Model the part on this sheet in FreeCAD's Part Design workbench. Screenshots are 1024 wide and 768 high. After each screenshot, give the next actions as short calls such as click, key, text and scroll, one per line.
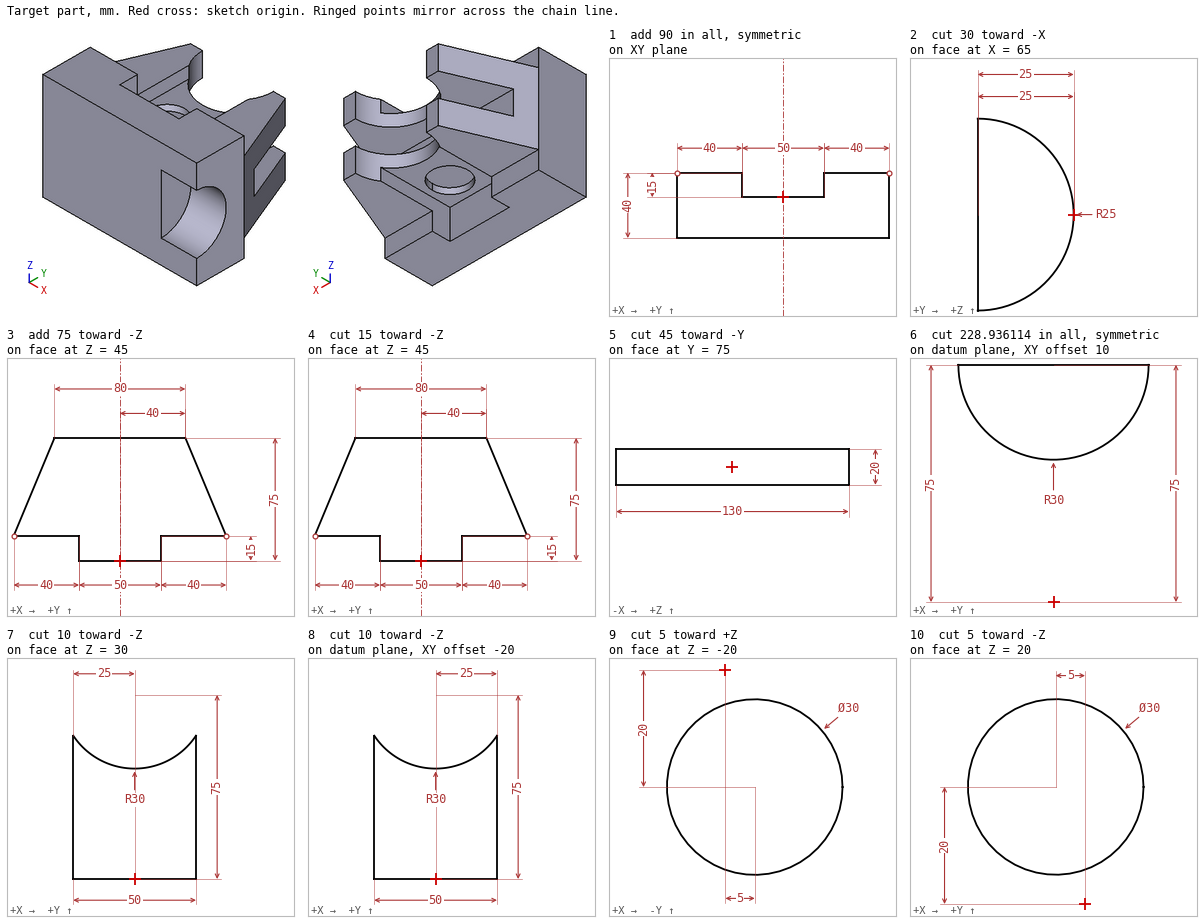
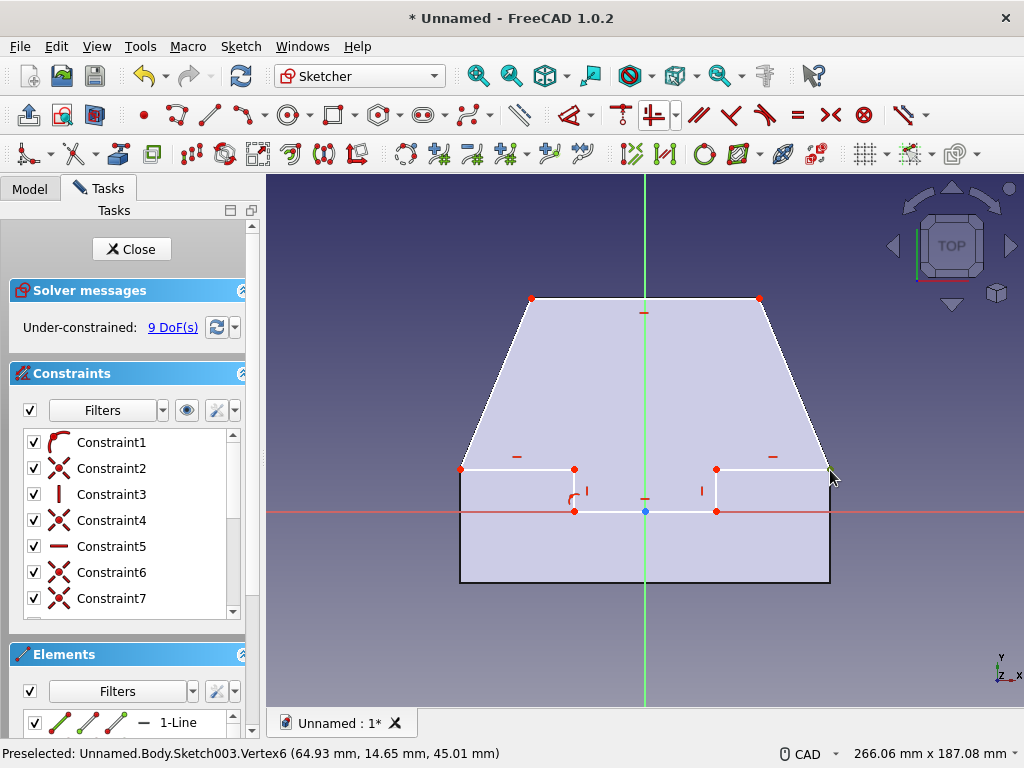
click(460, 470)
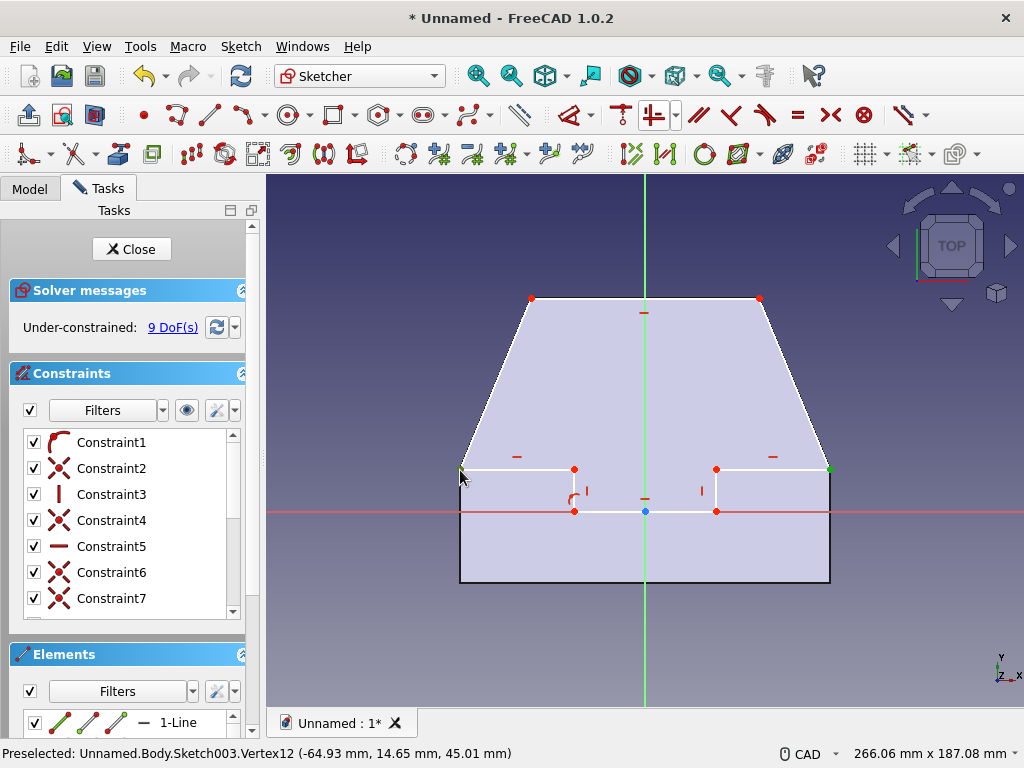
click(645, 645)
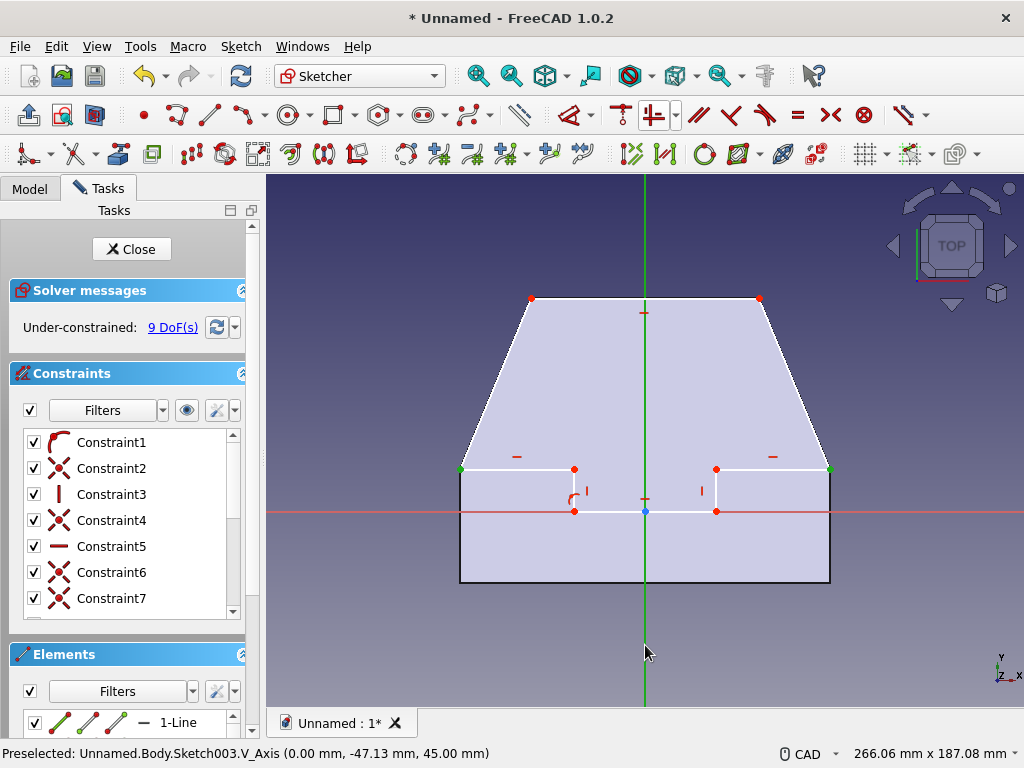
click(831, 116)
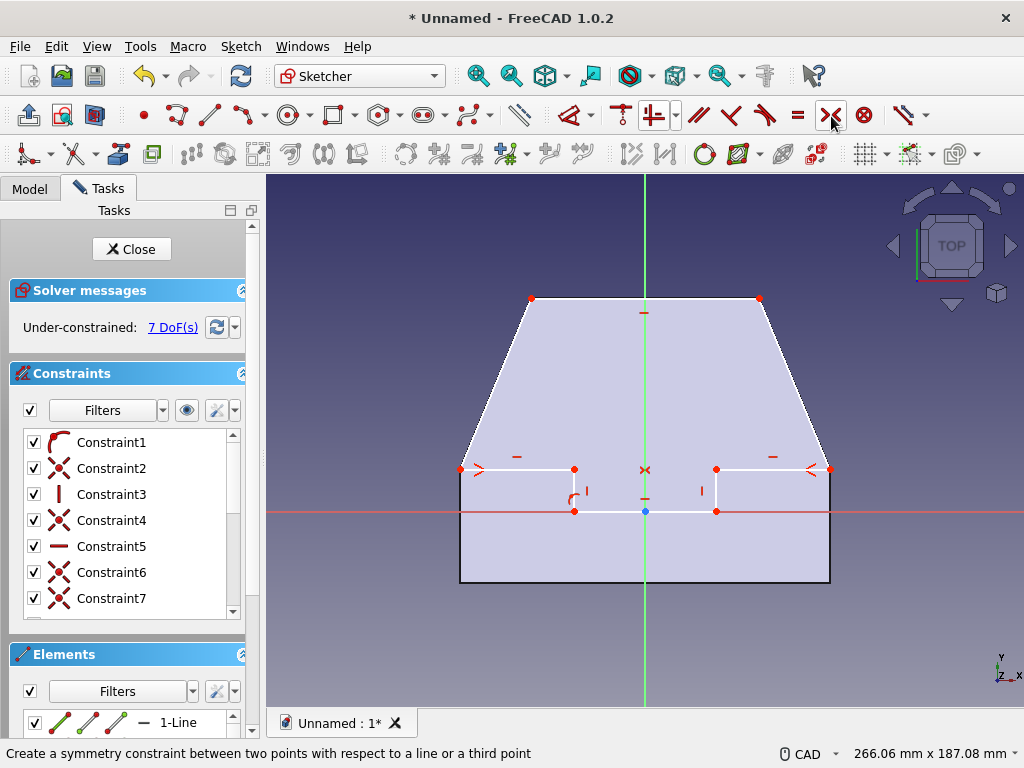
click(568, 116)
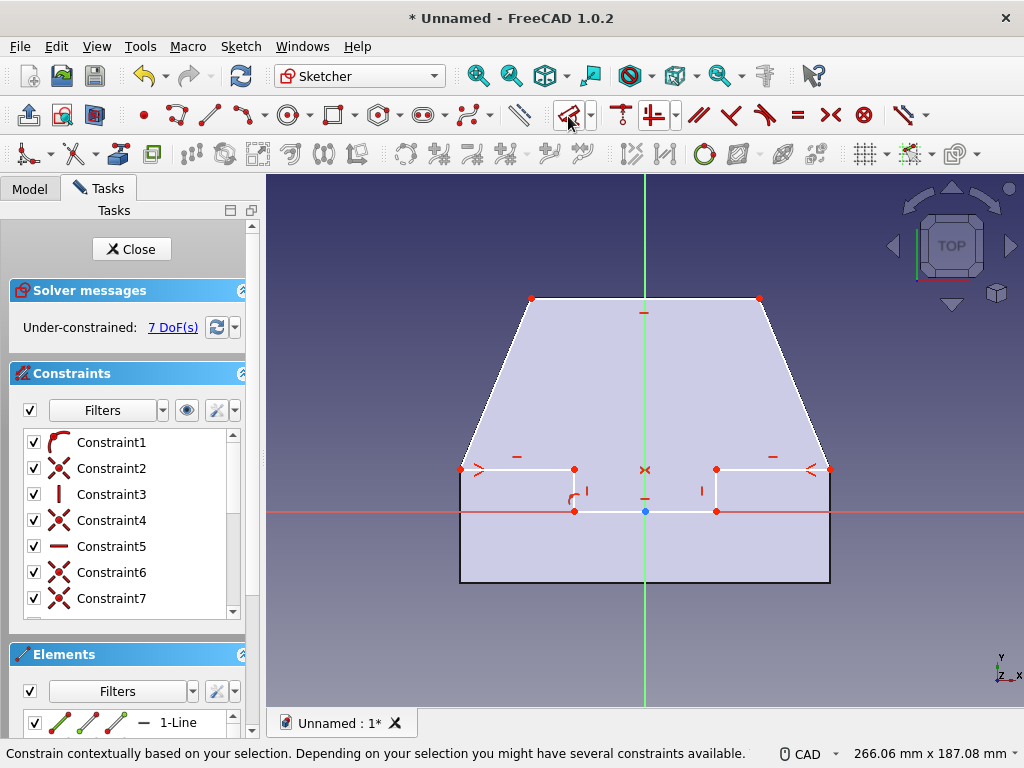
click(617, 512)
click(612, 546)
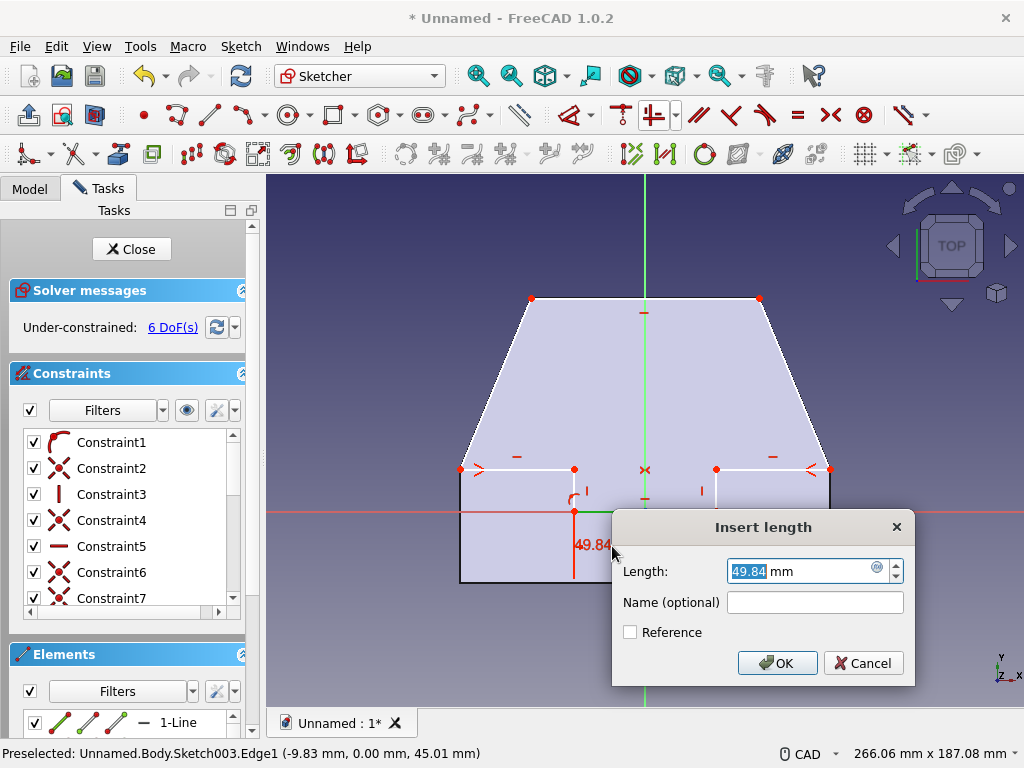
text(50)
key(Return)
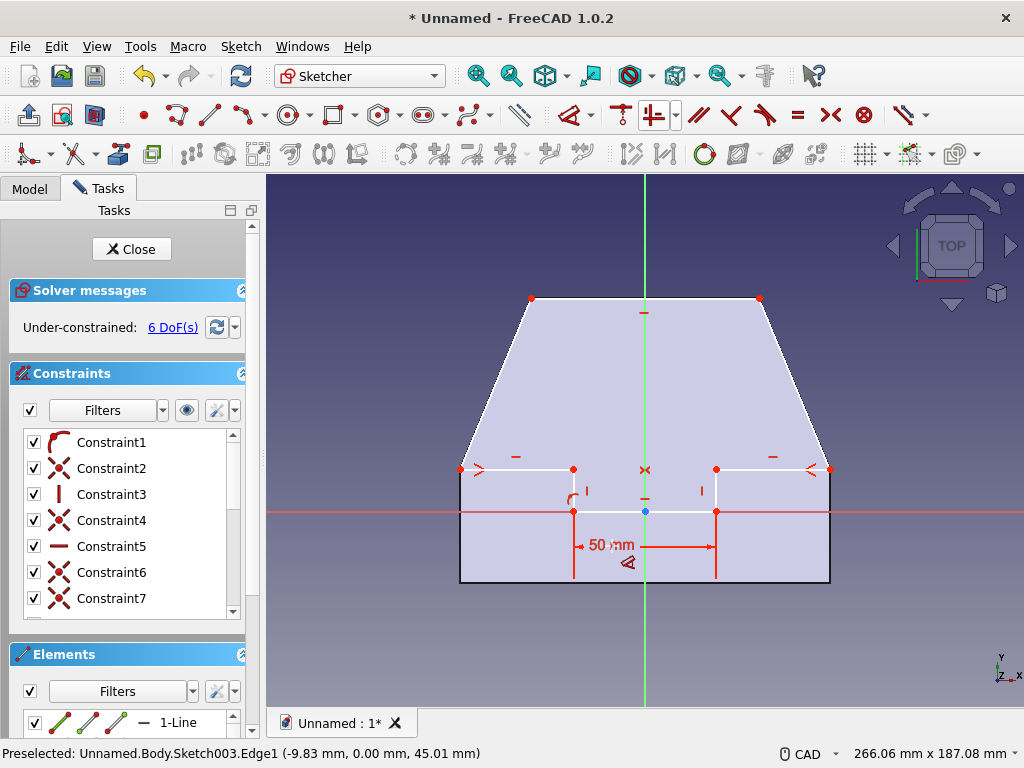
click(716, 499)
click(750, 491)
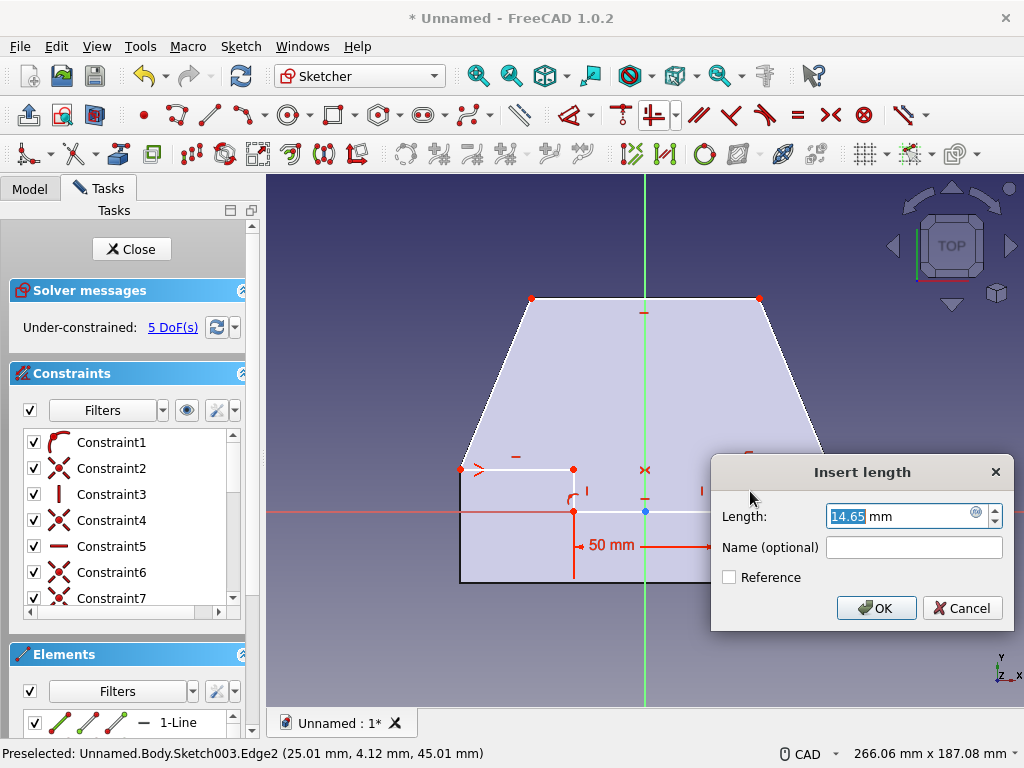
text(15)
key(Return)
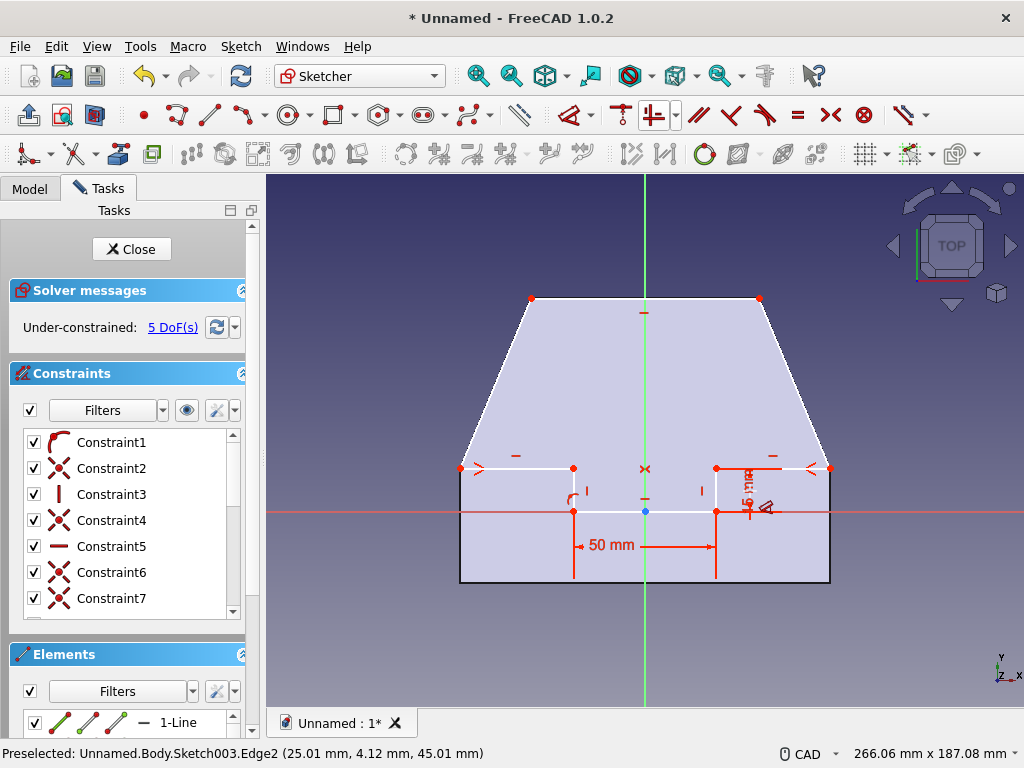
click(750, 469)
click(773, 435)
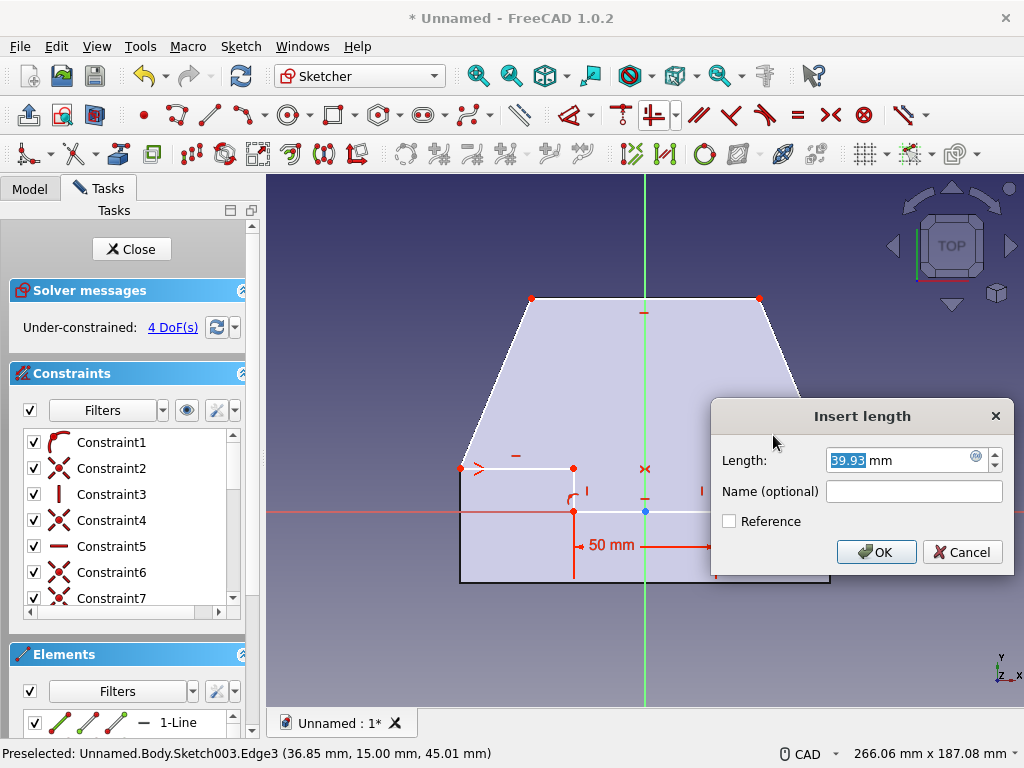
text(40)
key(Return)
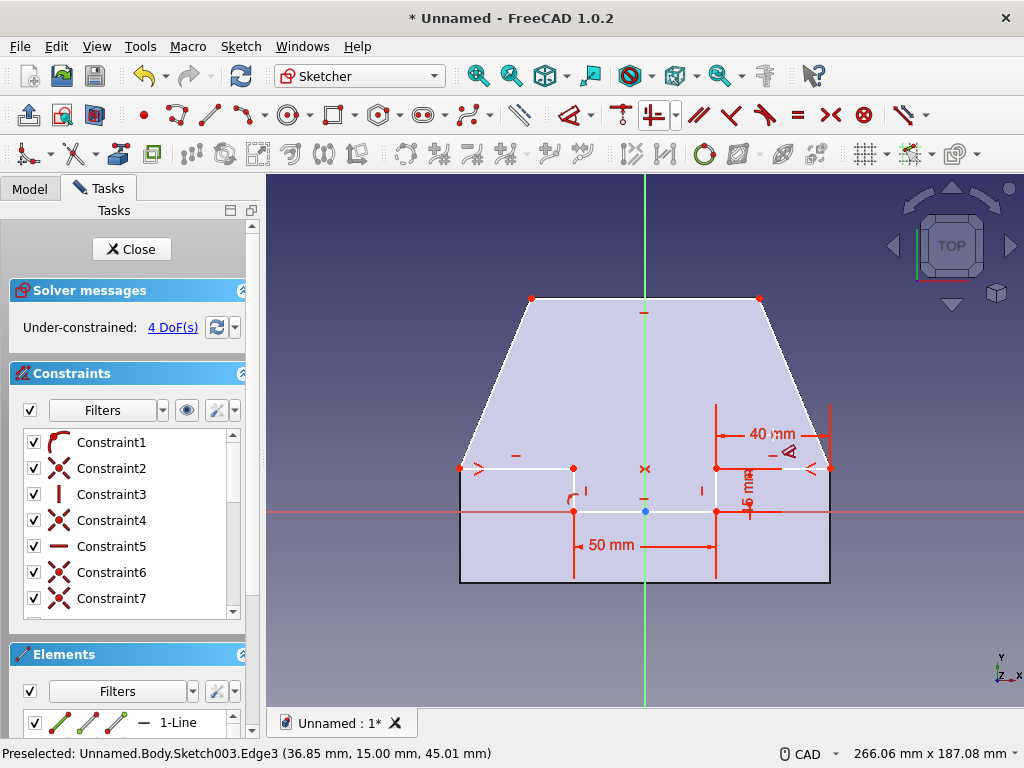
click(691, 299)
click(593, 265)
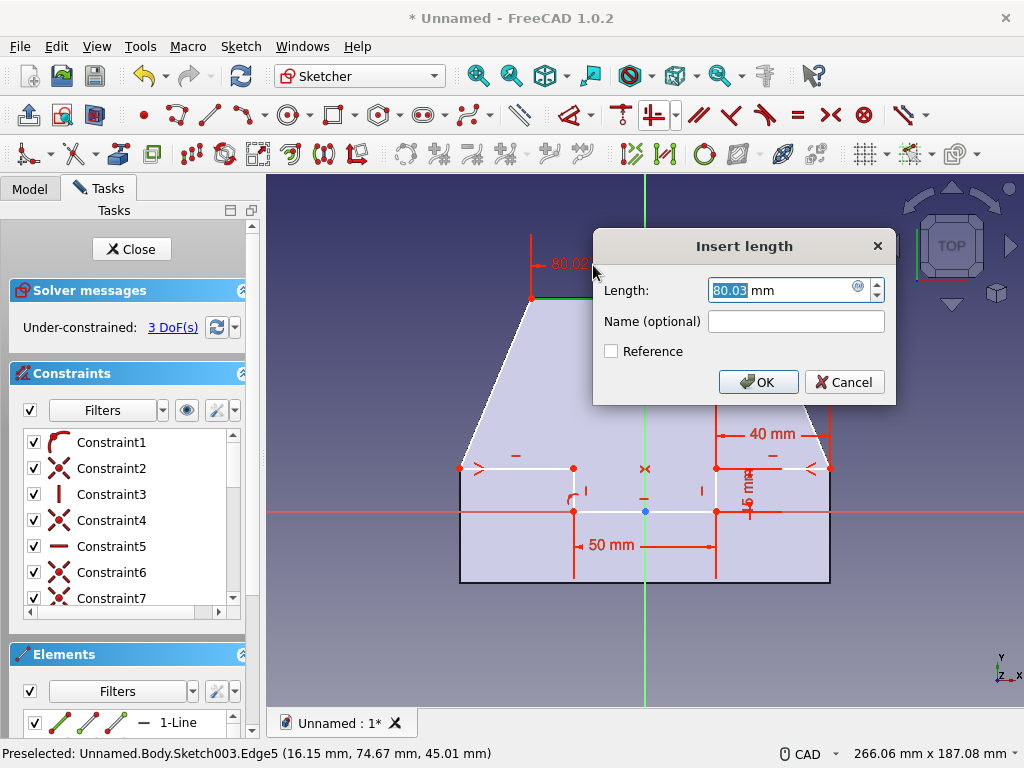
text(80)
key(Return)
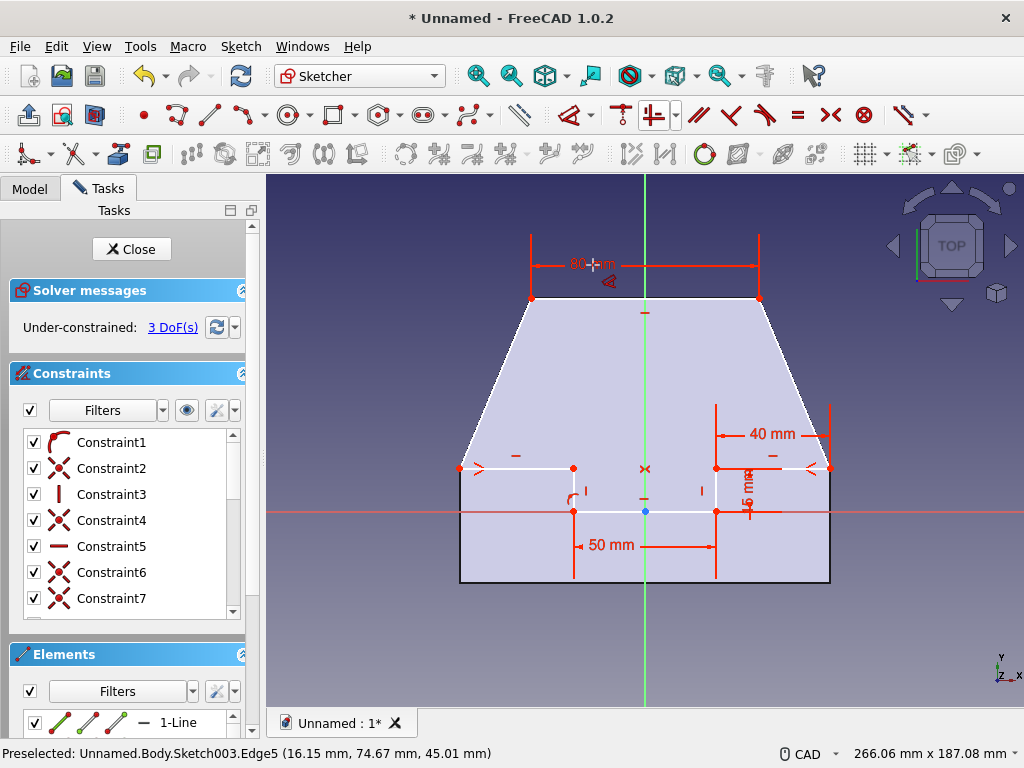
click(494, 469)
click(517, 435)